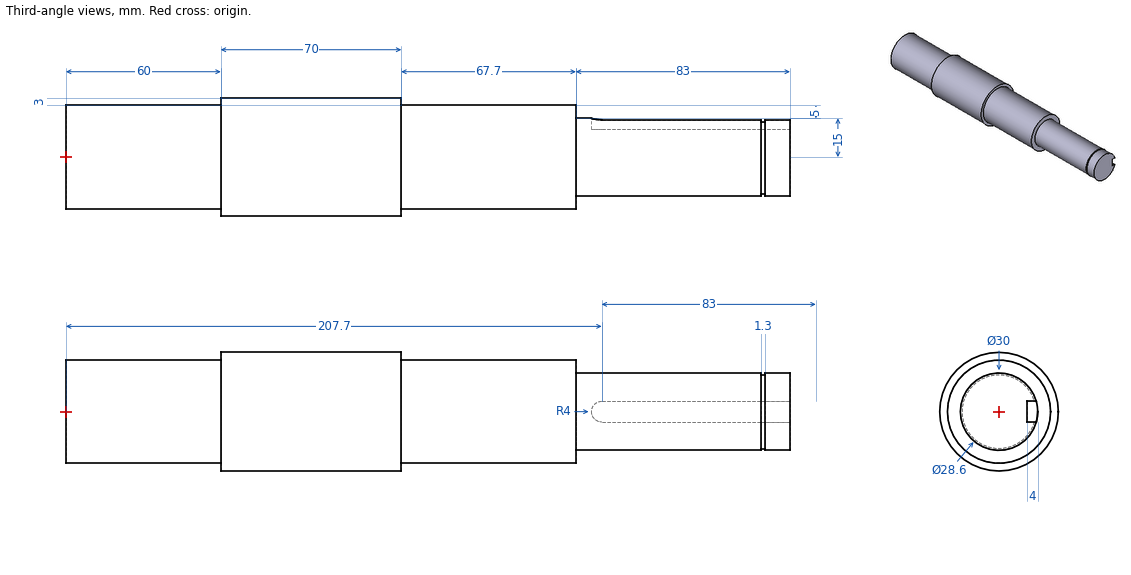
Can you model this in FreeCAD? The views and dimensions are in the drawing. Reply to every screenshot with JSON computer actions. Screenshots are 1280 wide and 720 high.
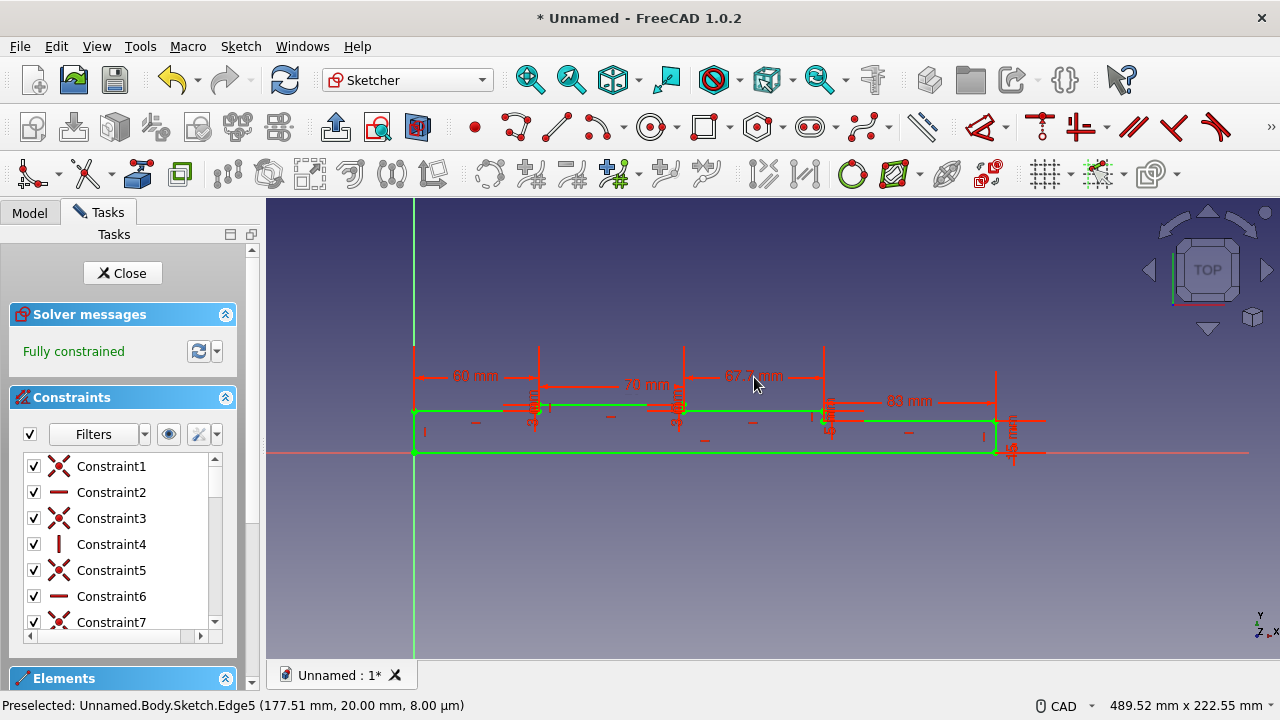
{"action": "left_click", "coordinate": [123, 273]}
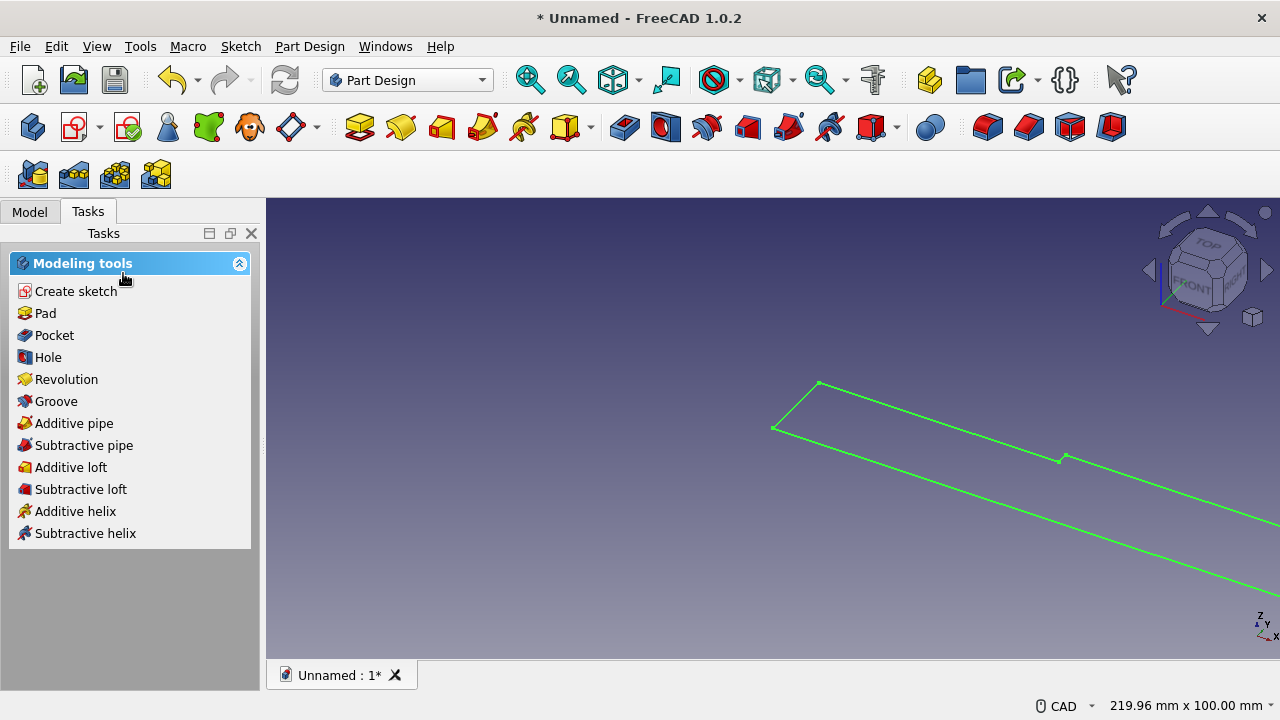
{"action": "left_click", "coordinate": [401, 128]}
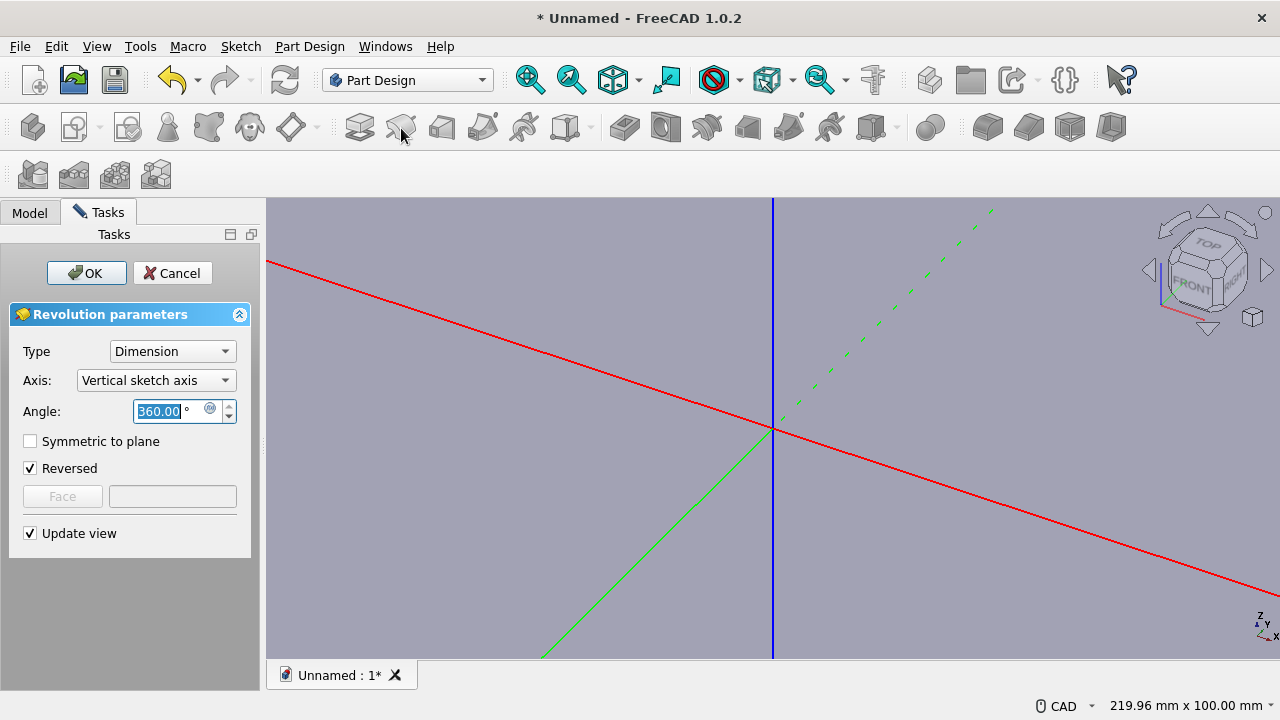
{"action": "left_click", "coordinate": [157, 380]}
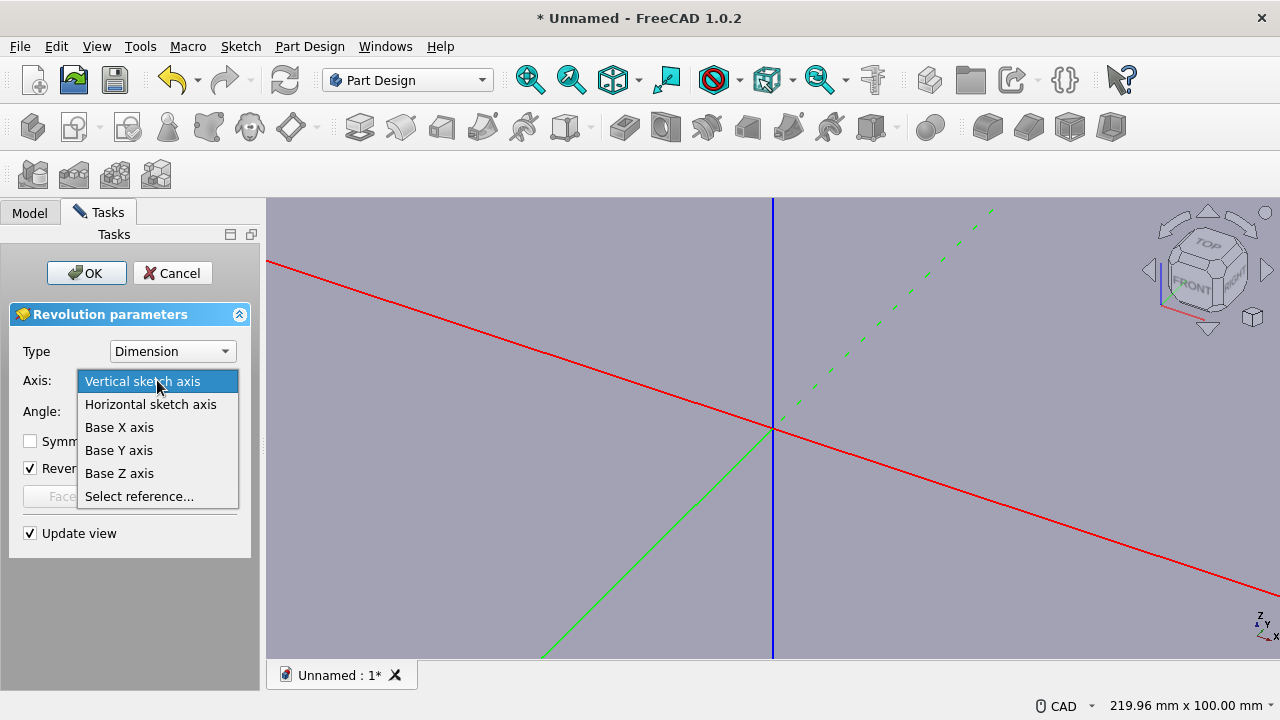
{"action": "left_click", "coordinate": [156, 404]}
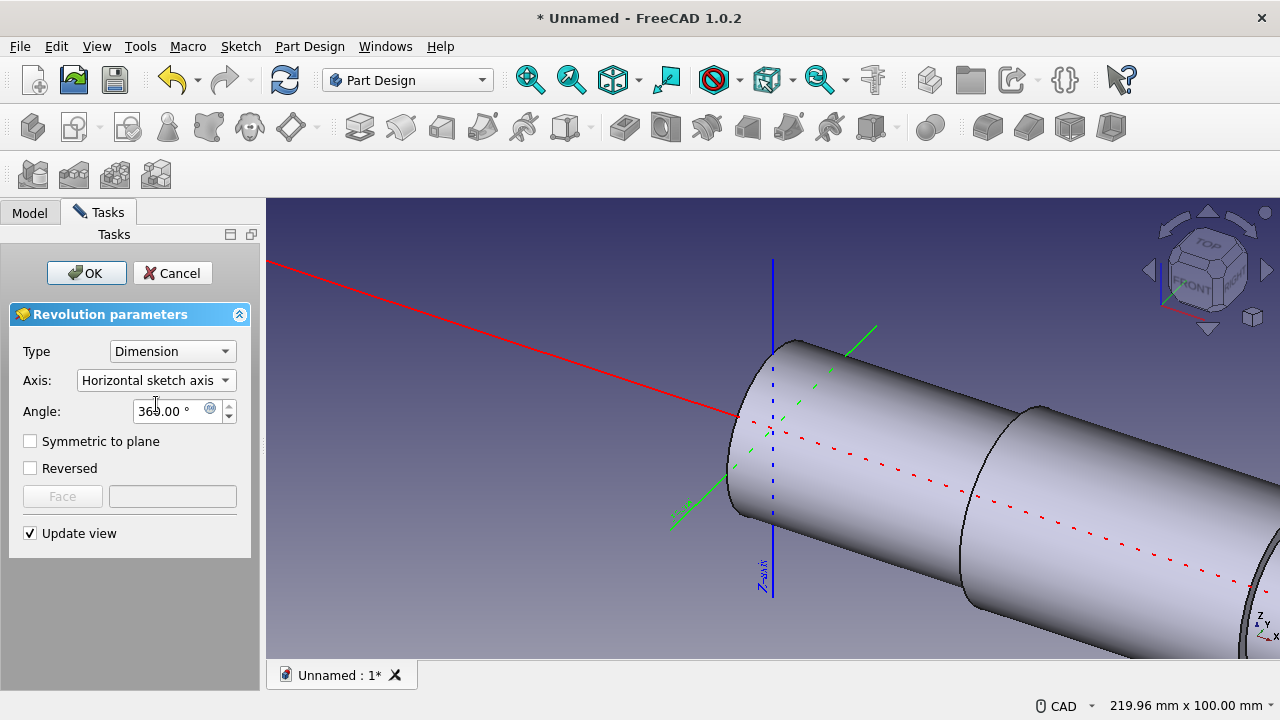
{"action": "left_click", "coordinate": [87, 273]}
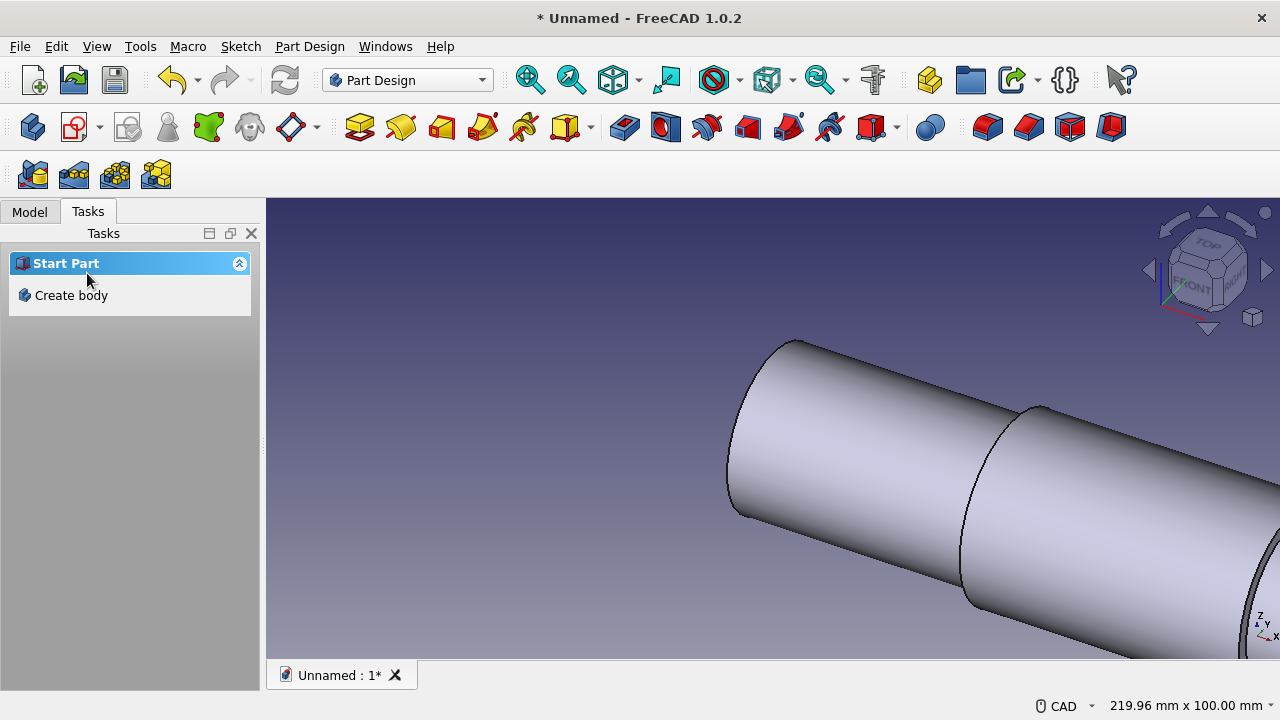
{"action": "key", "text": "v f"}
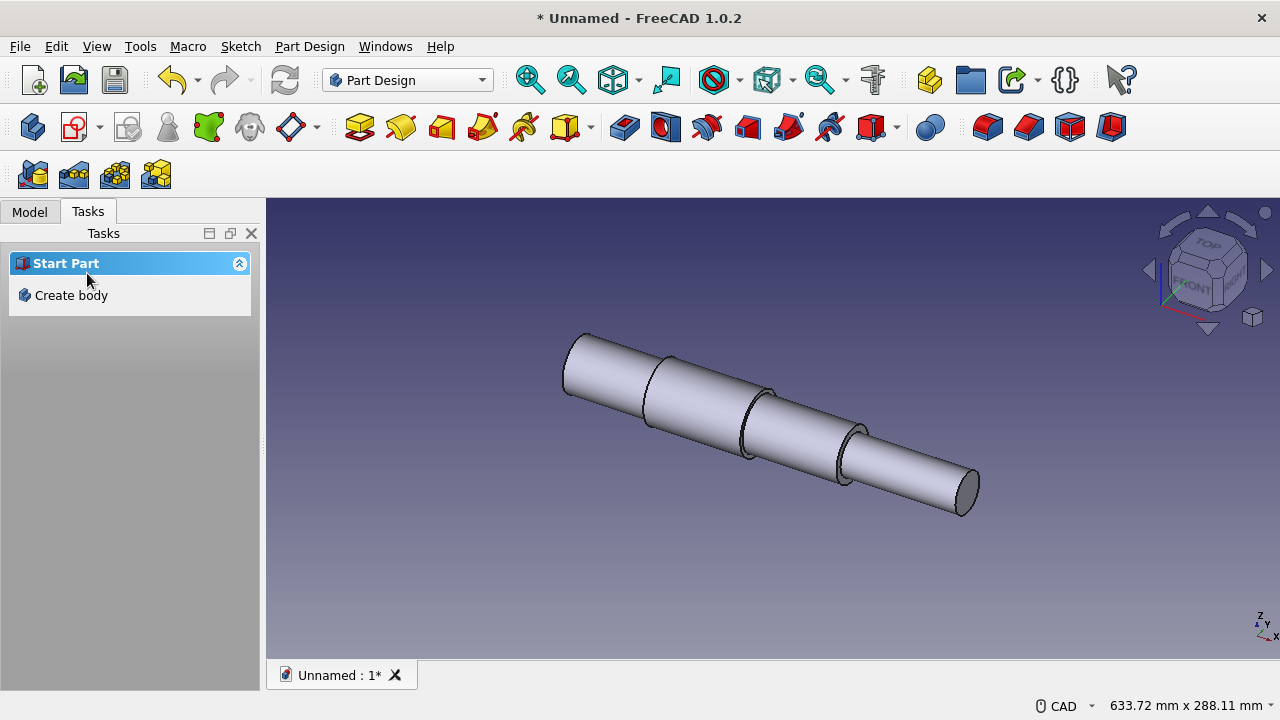
{"action": "left_click", "coordinate": [30, 212]}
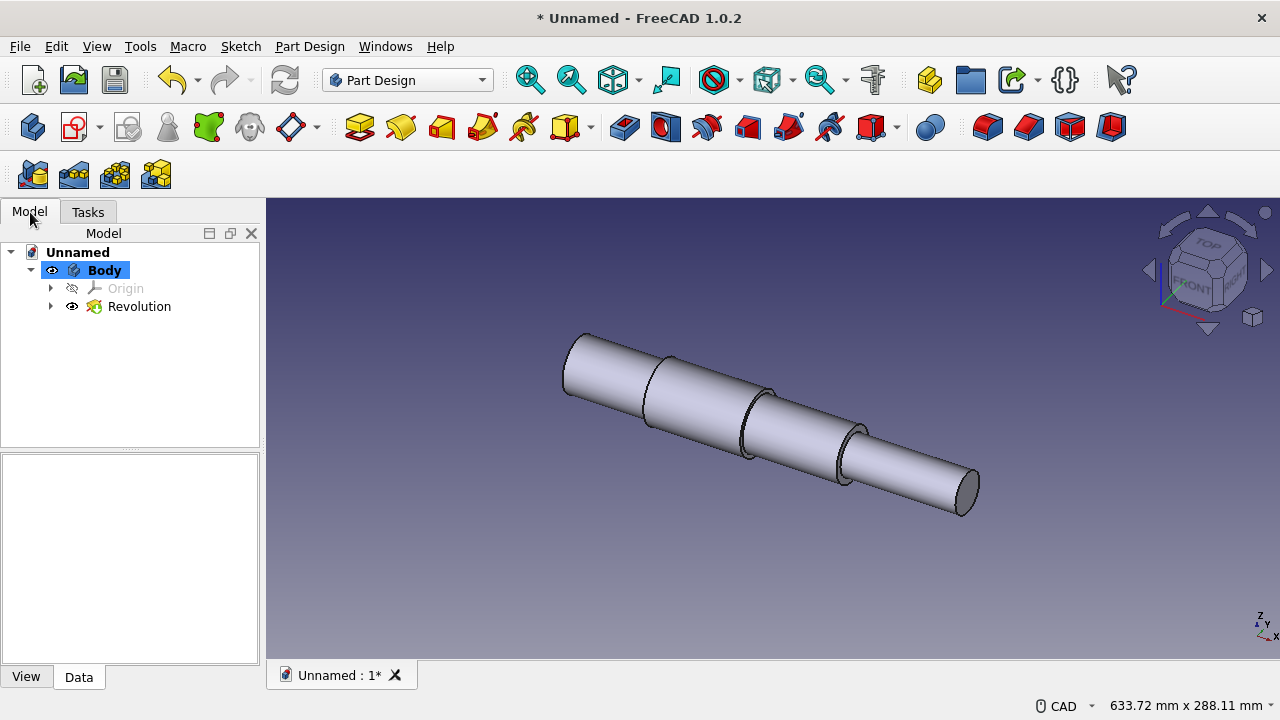
{"action": "left_click", "coordinate": [51, 288]}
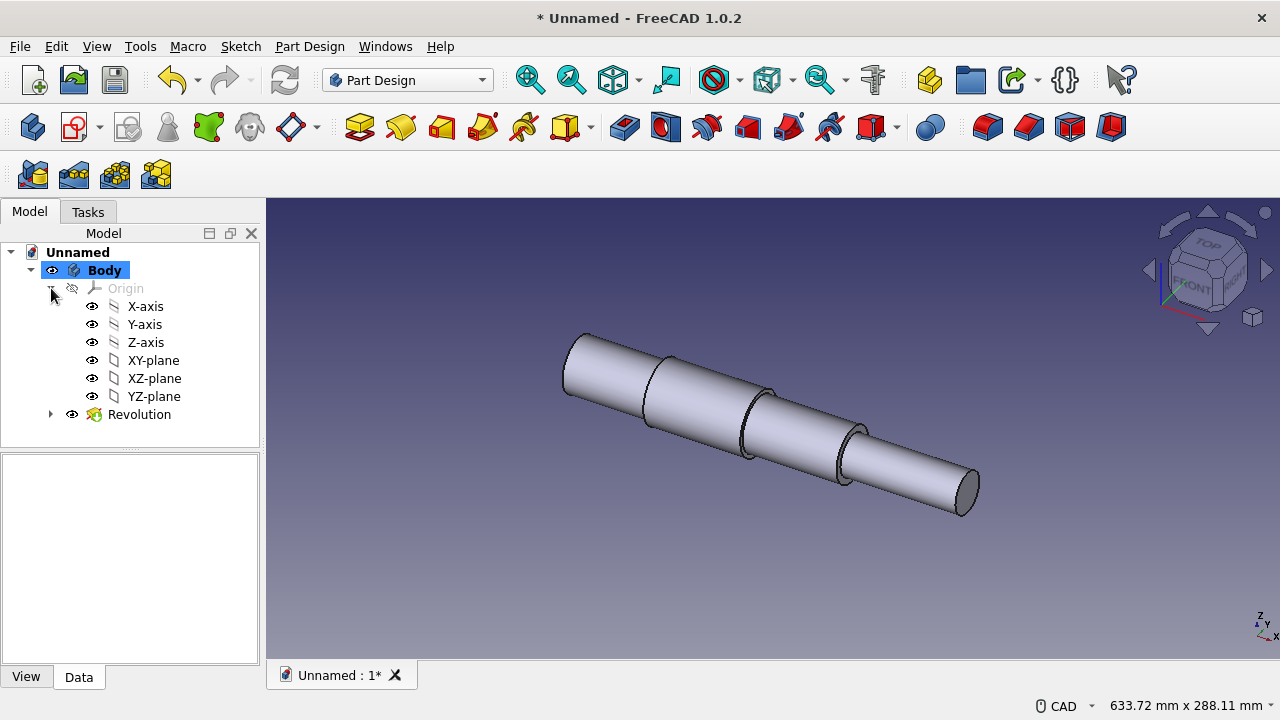
{"action": "left_click", "coordinate": [137, 378]}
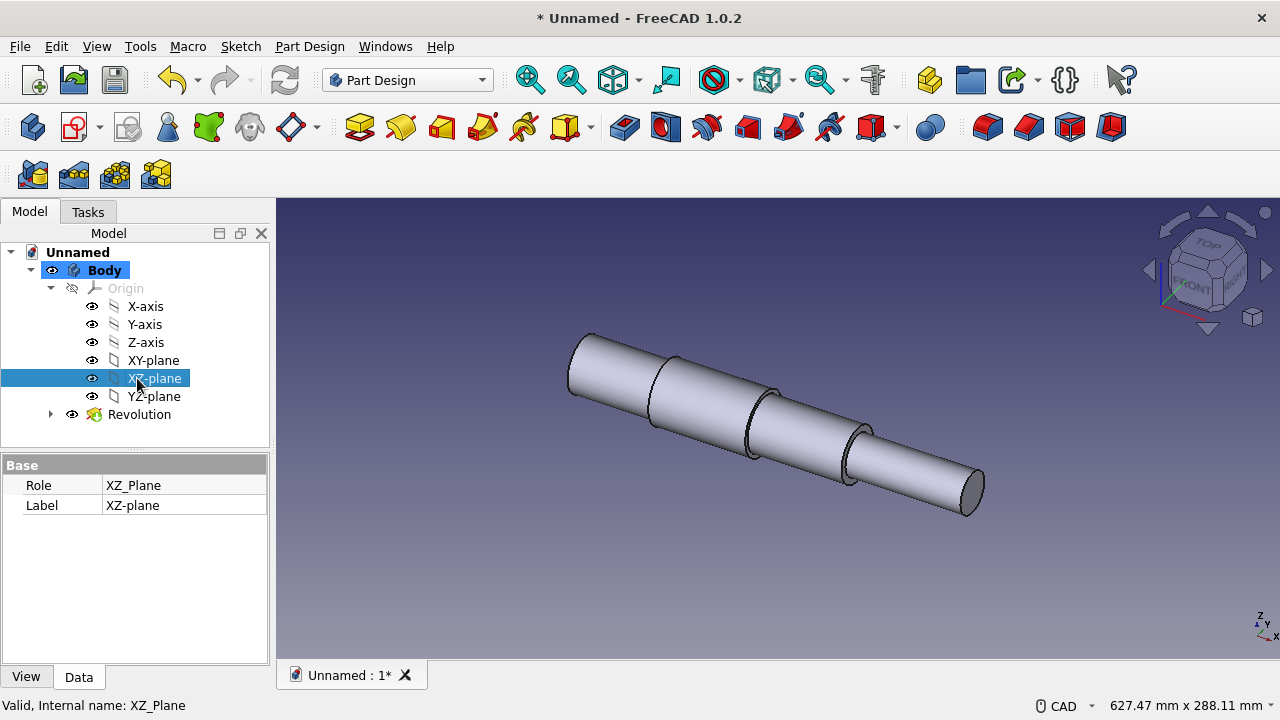
{"action": "left_click", "coordinate": [290, 128]}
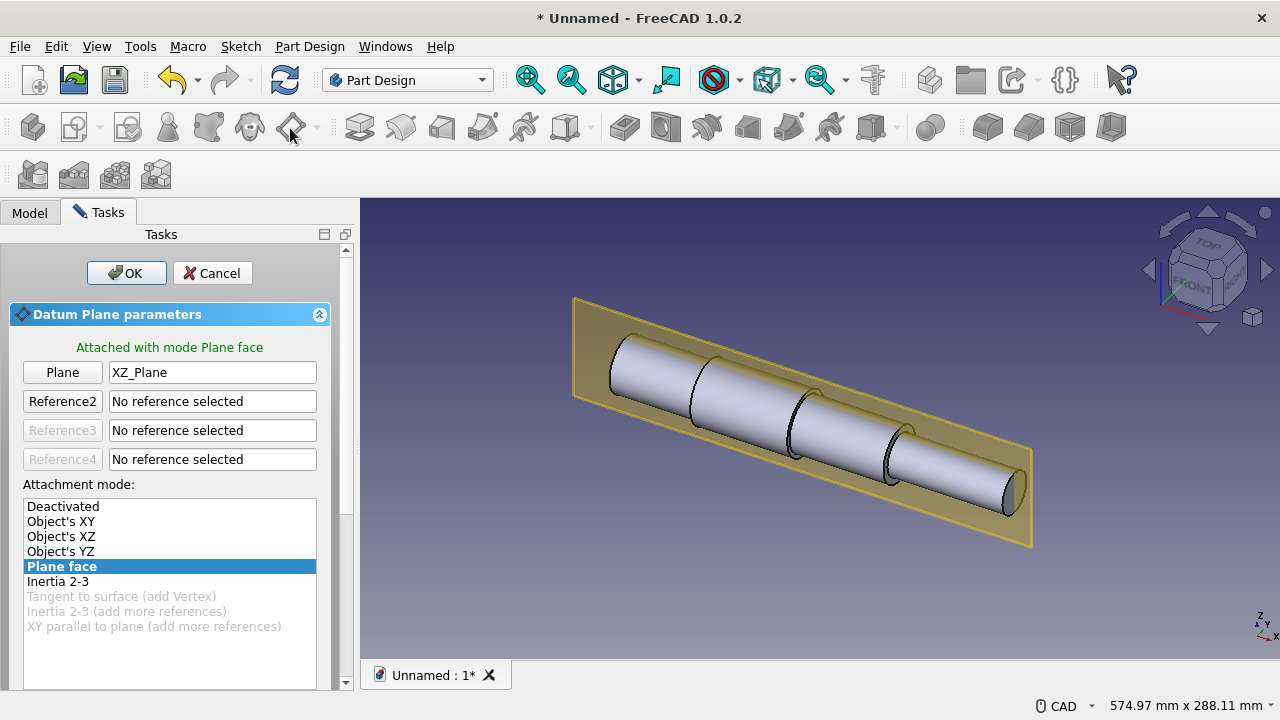
{"action": "scroll", "coordinate": [346, 467], "scroll_direction": "down", "scroll_amount": 4}